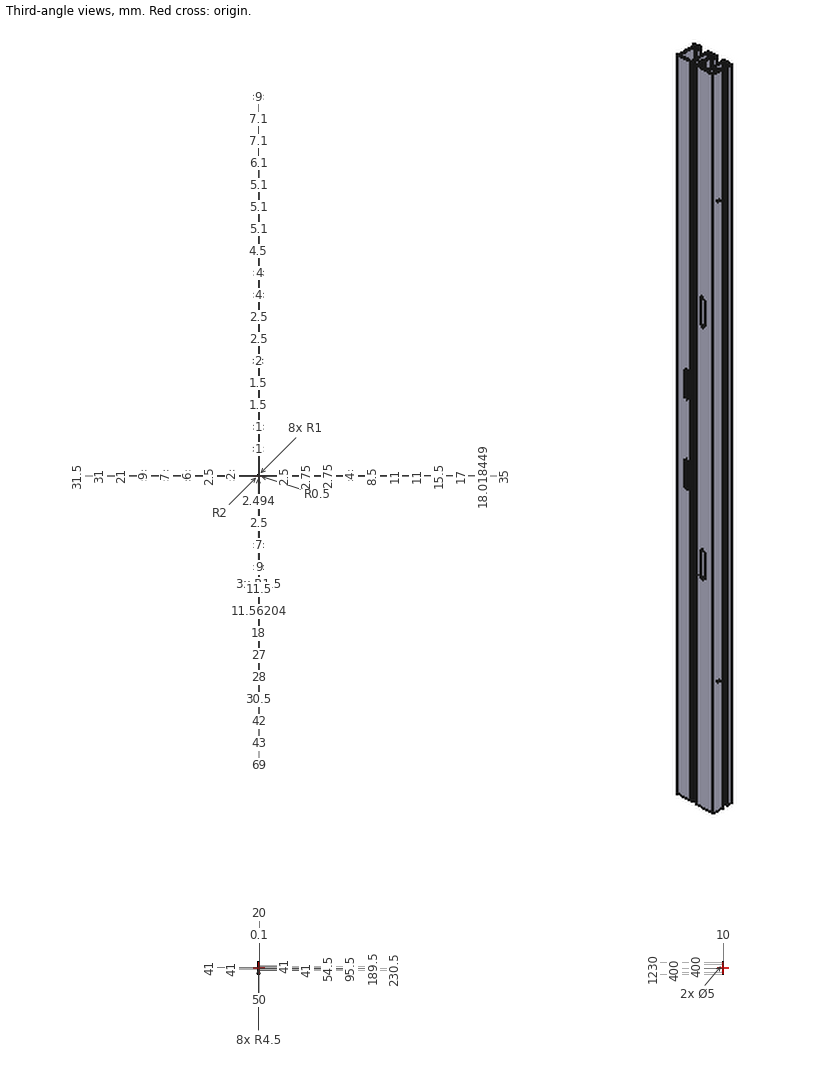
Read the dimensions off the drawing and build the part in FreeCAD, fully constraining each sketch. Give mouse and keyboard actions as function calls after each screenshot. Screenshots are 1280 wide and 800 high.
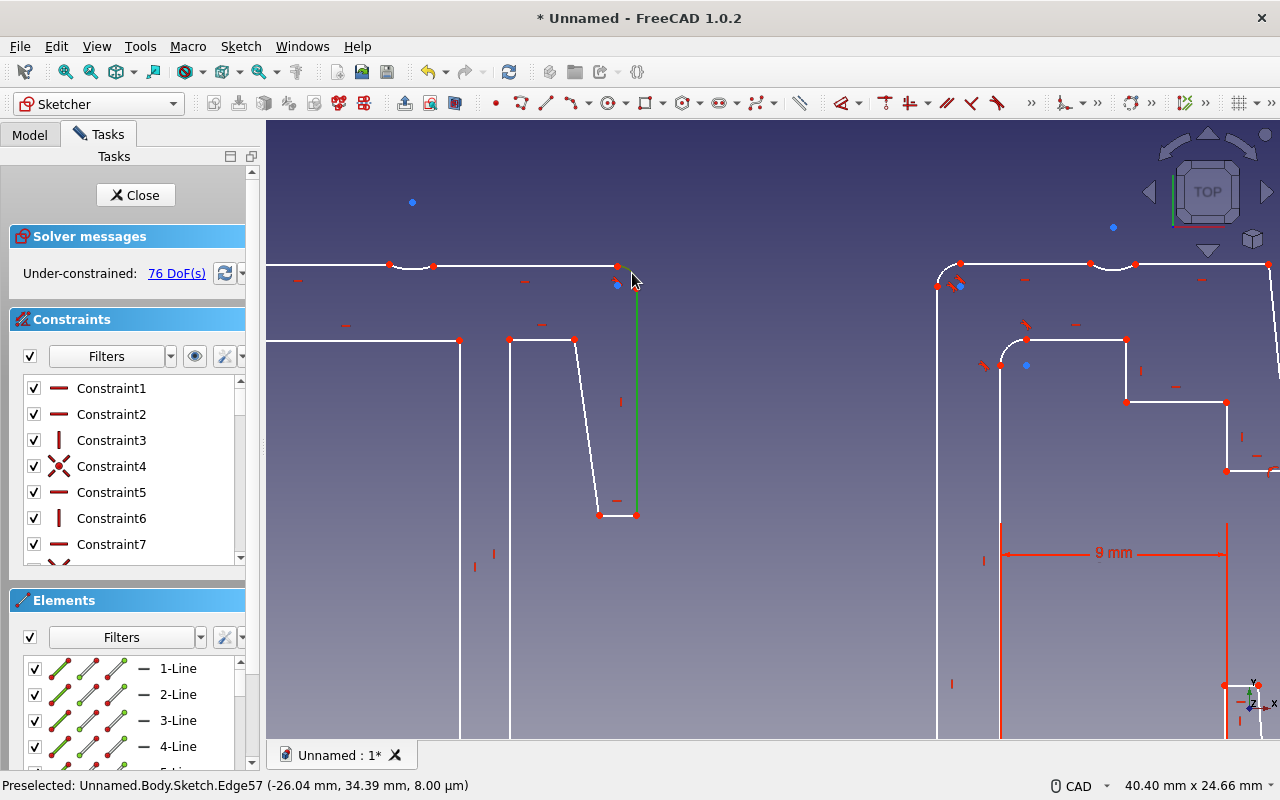
click(997, 104)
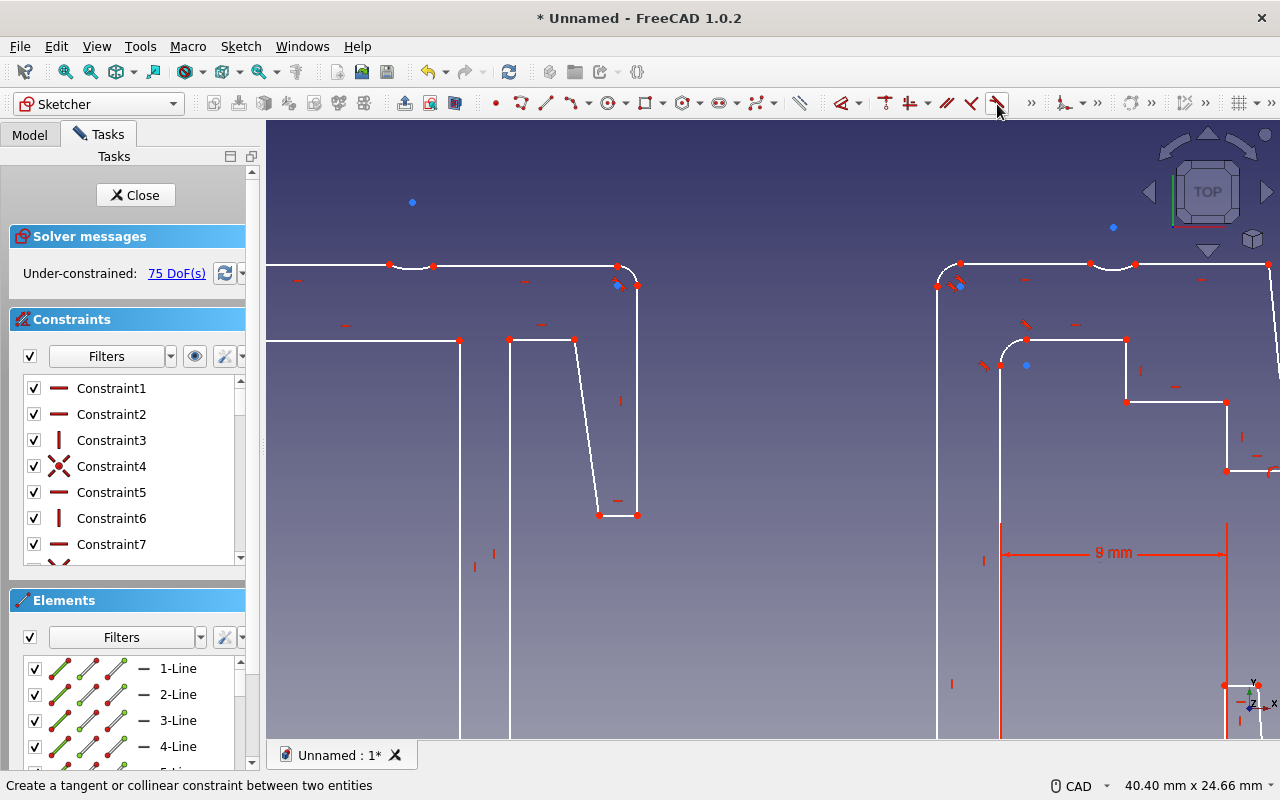
scroll(831, 312, down, 6)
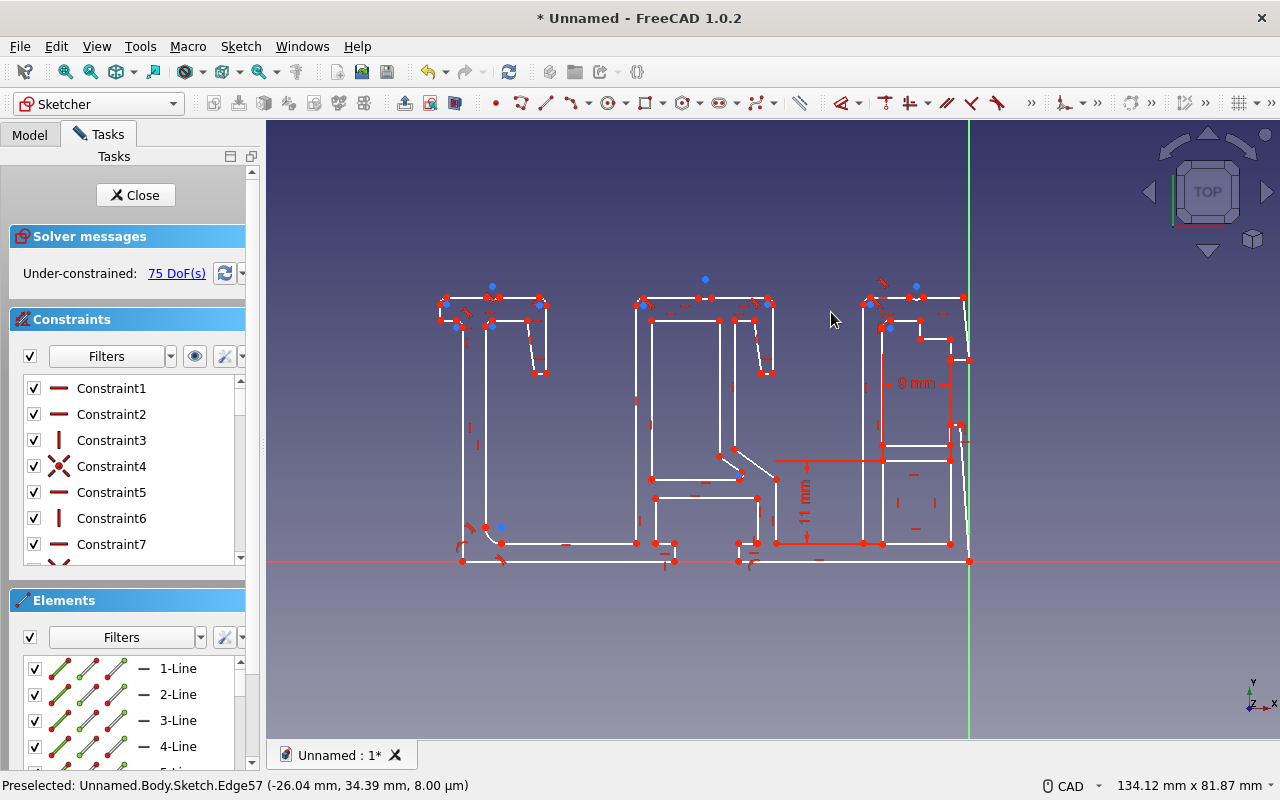
click(713, 480)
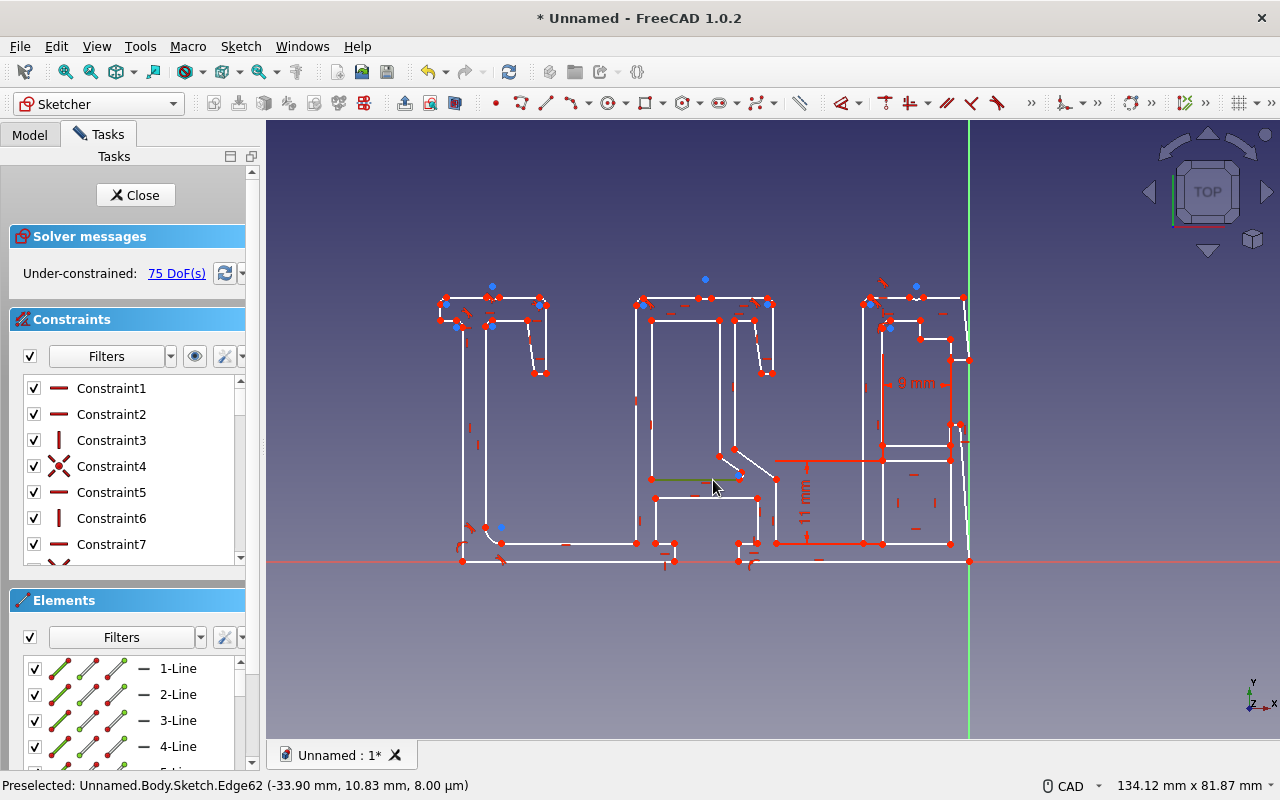
scroll(743, 477, up, 6)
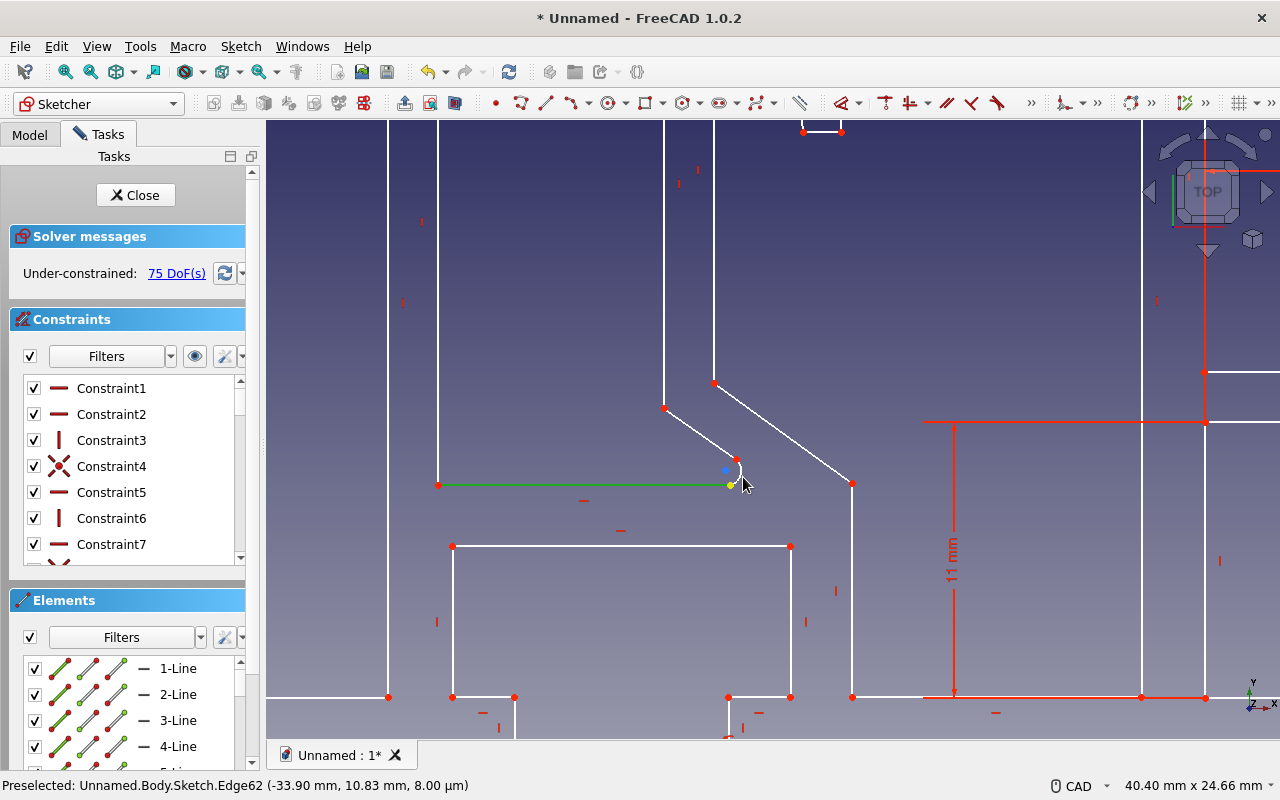
click(741, 474)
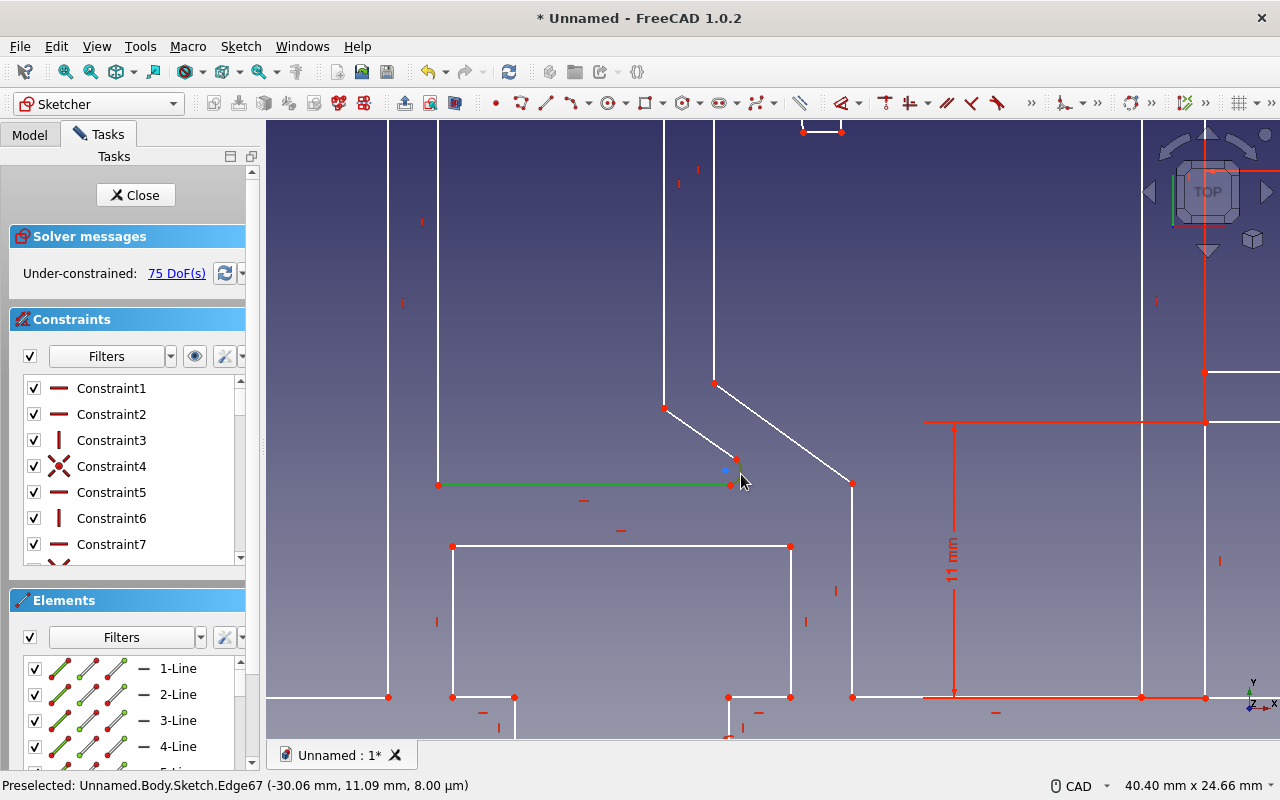
click(997, 104)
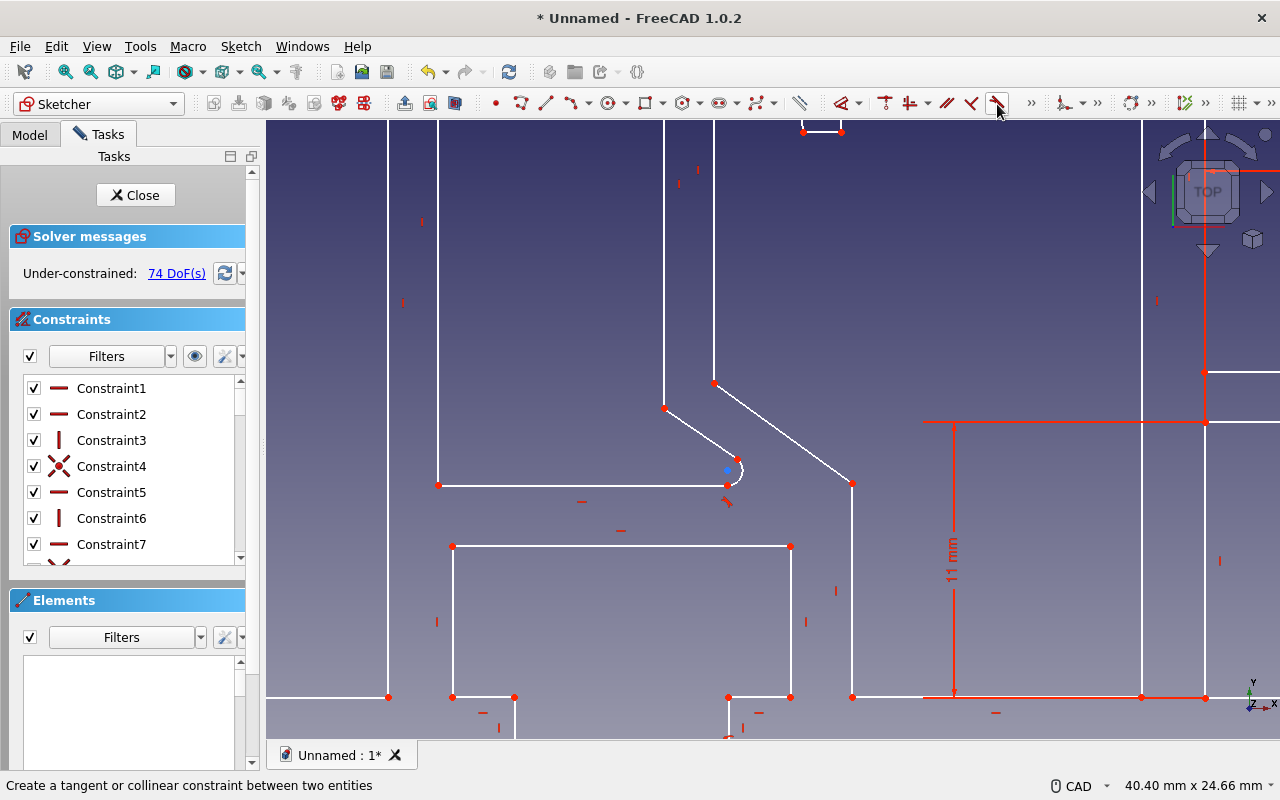
click(686, 424)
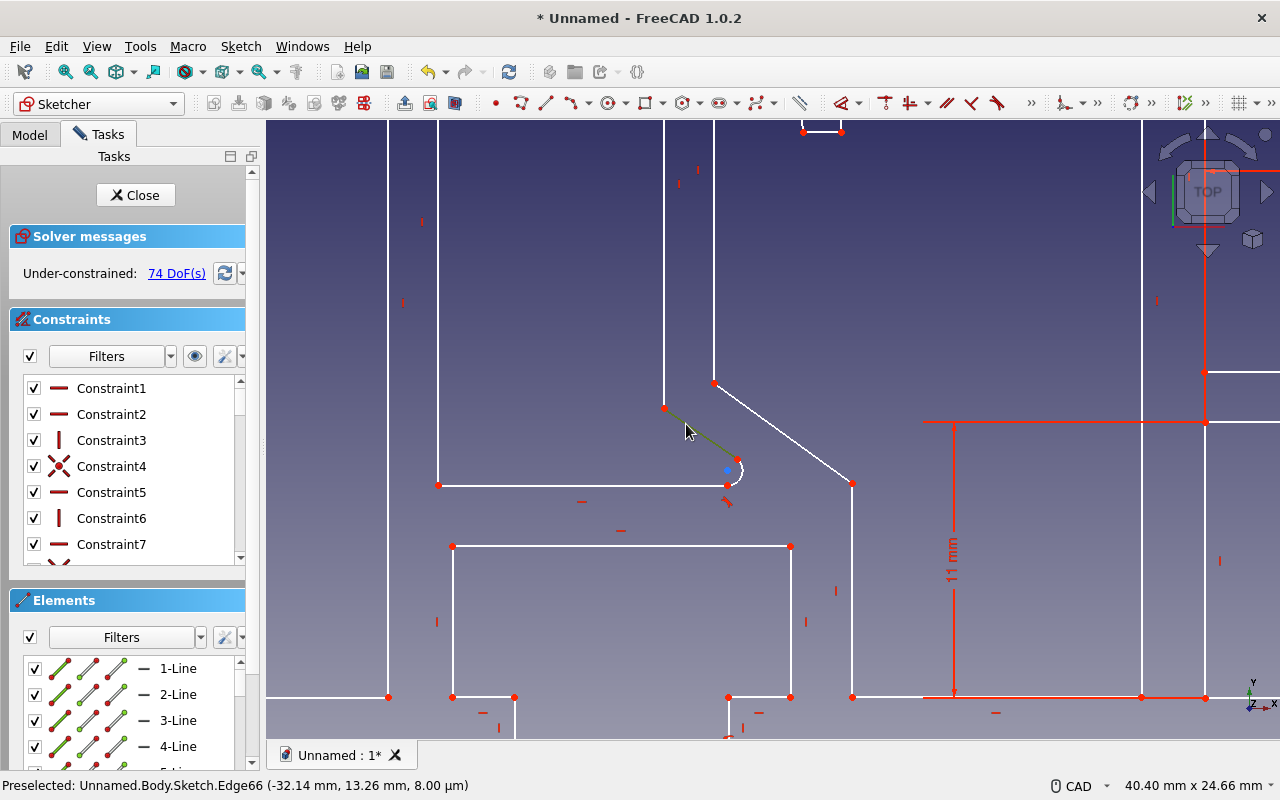
scroll(737, 482, up, 2)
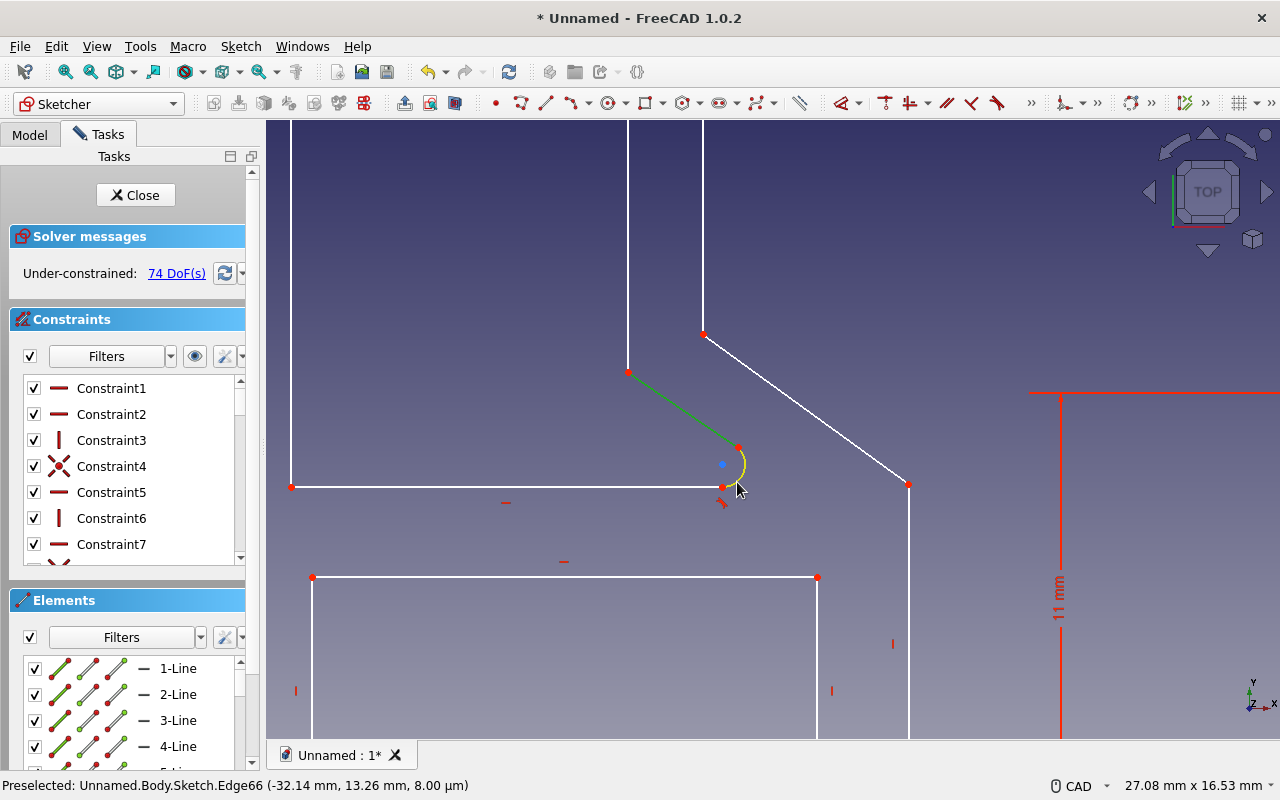
click(737, 482)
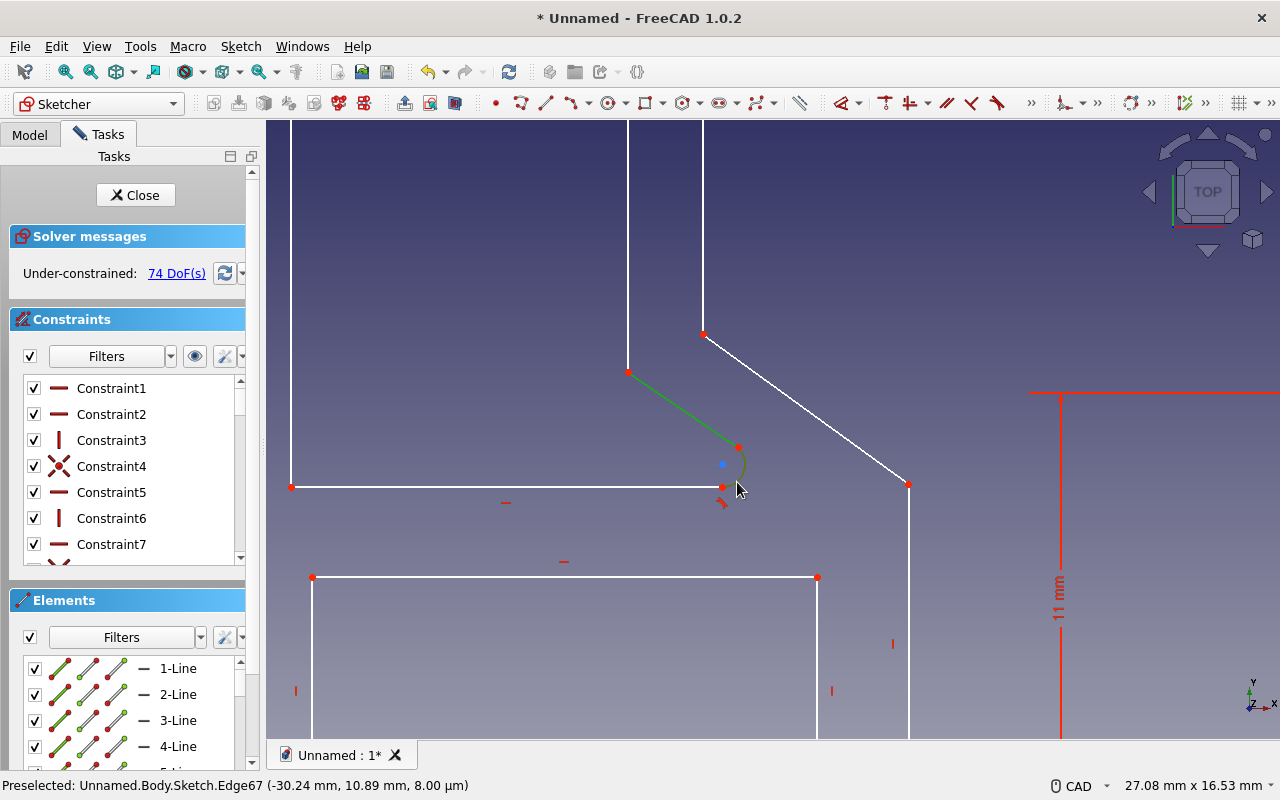
click(997, 104)